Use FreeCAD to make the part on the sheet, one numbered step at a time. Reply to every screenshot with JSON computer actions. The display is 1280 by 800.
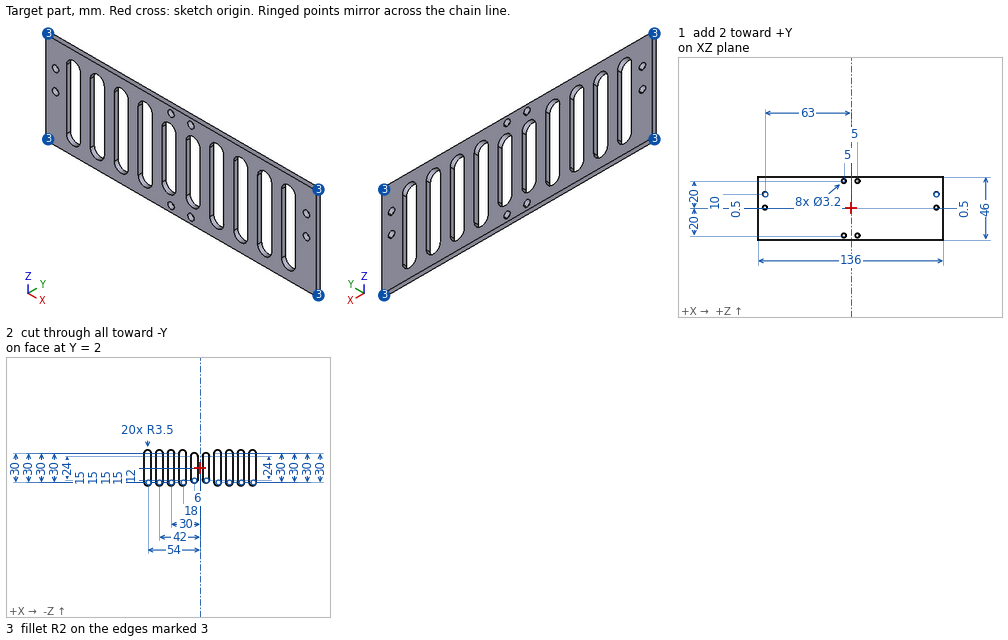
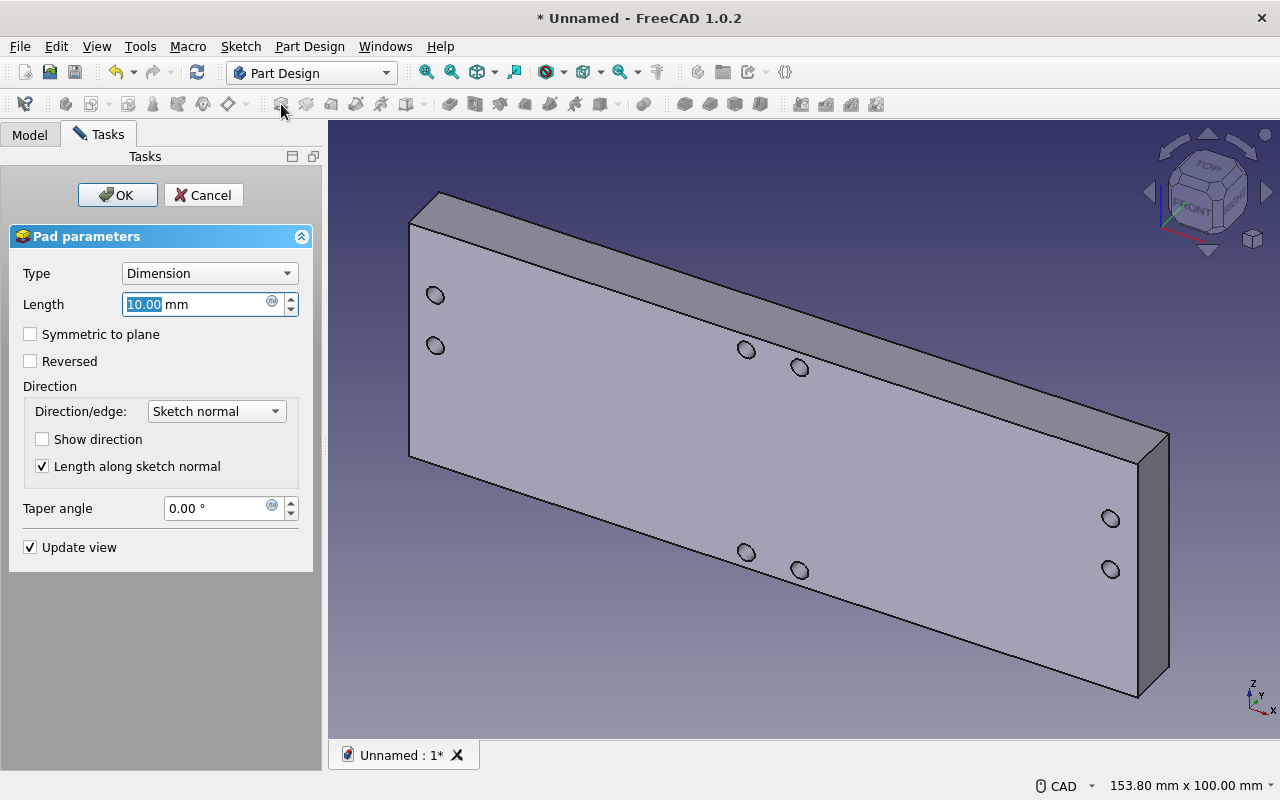
{"action": "type", "text": "2"}
{"action": "key", "text": "Tab"}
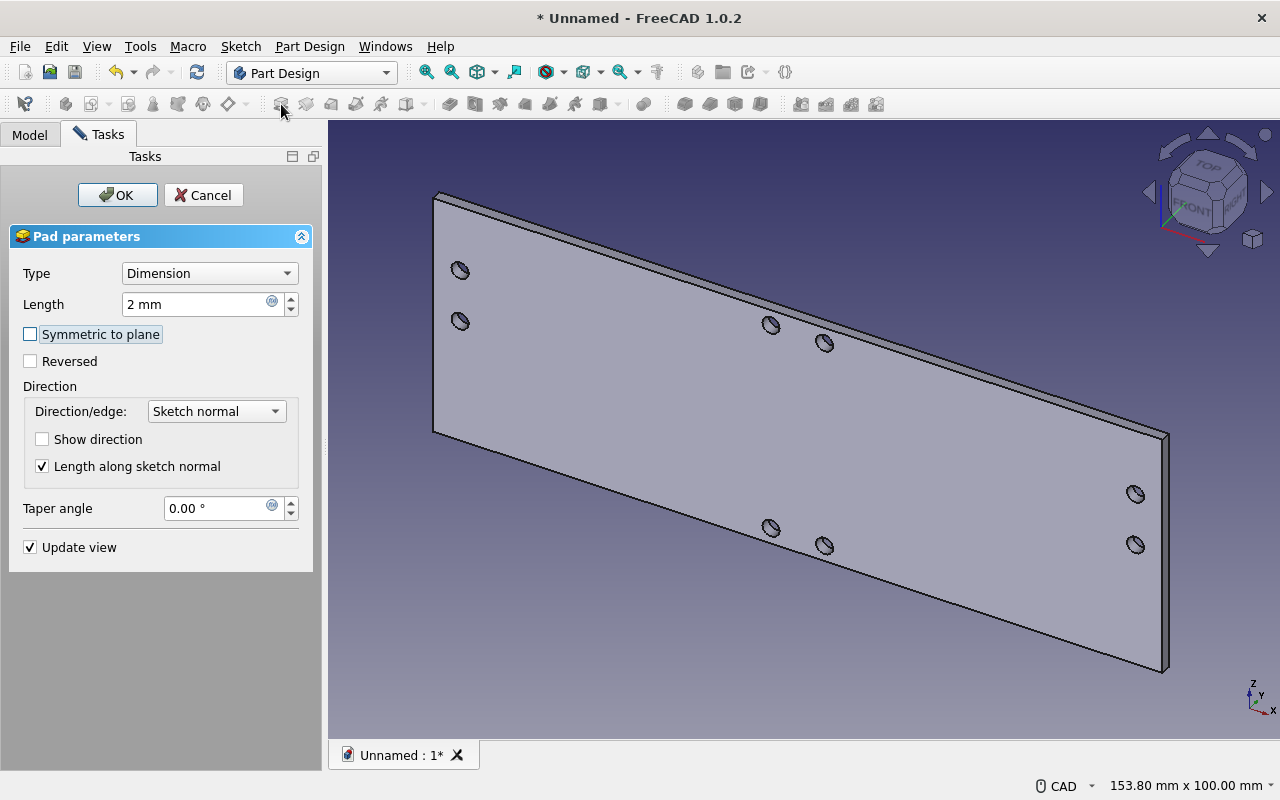
{"action": "left_click", "coordinate": [31, 361]}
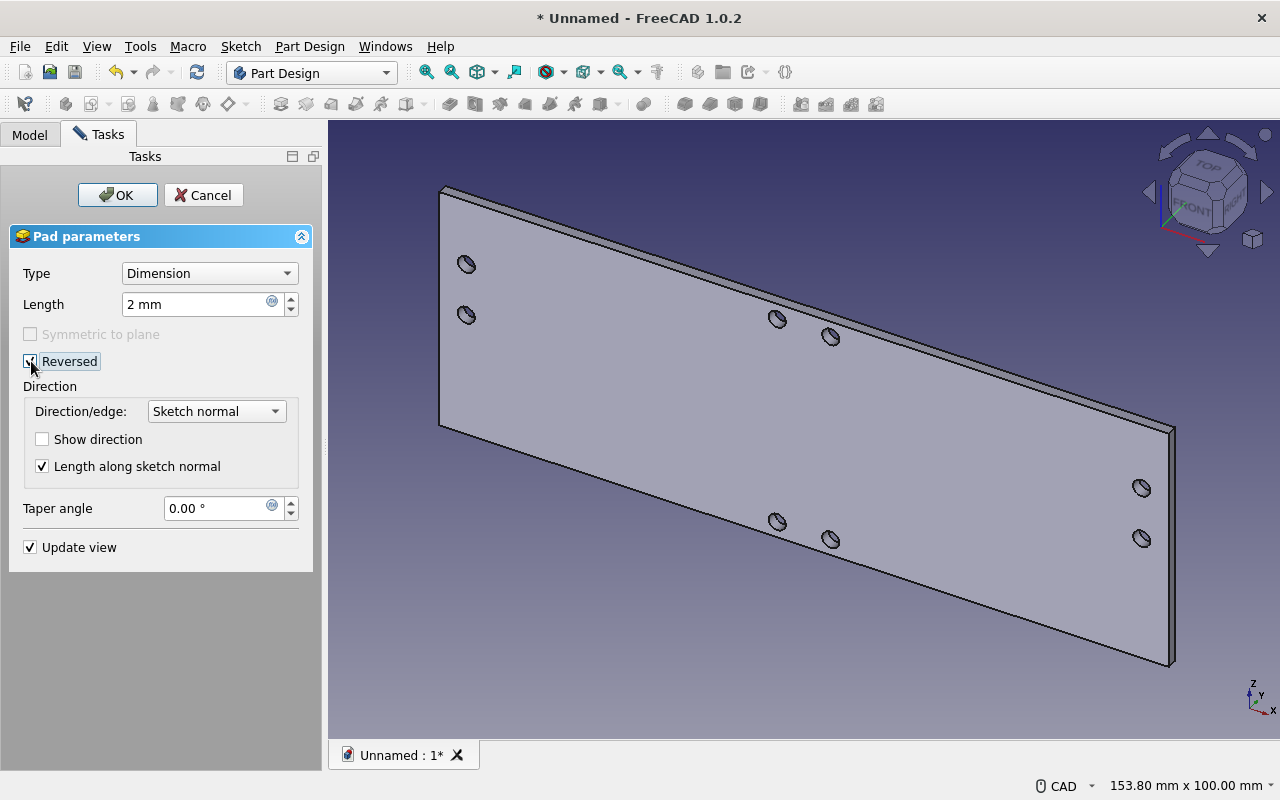
{"action": "left_click", "coordinate": [118, 195]}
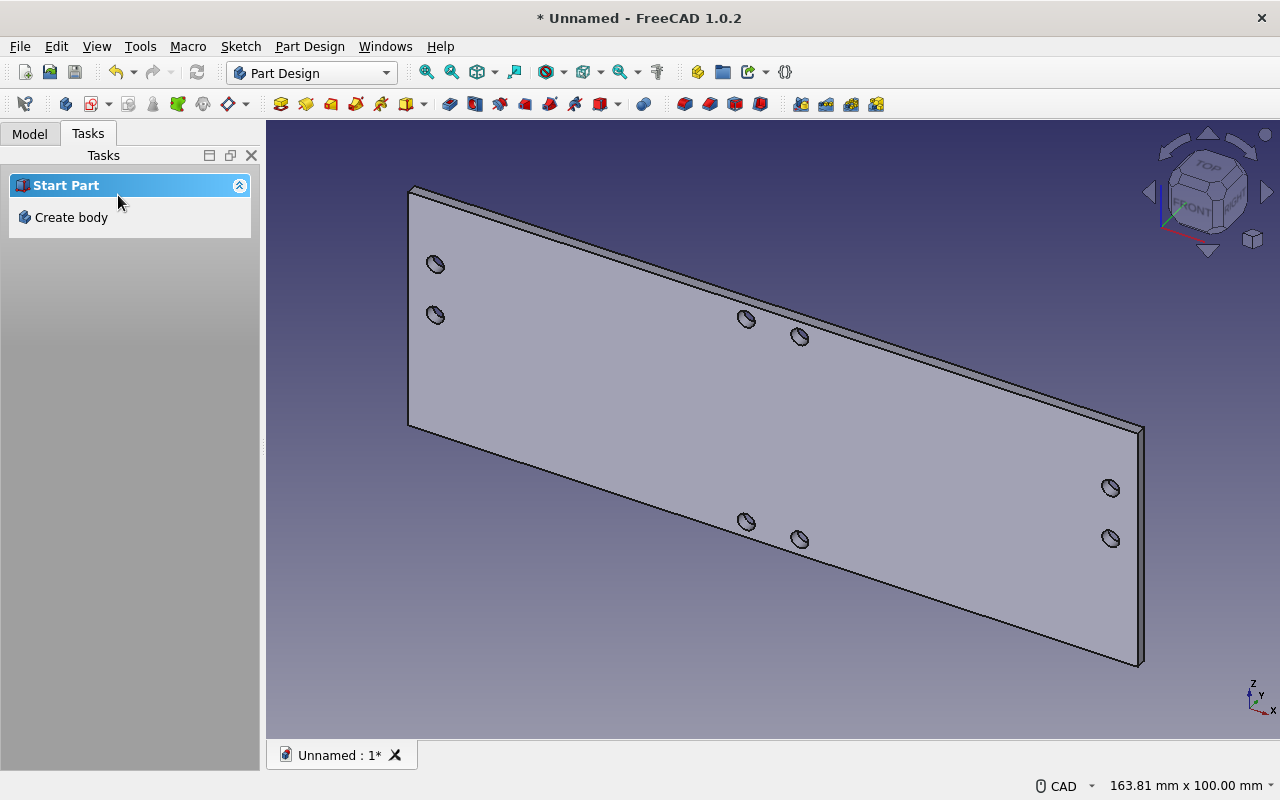
{"action": "key", "text": "4"}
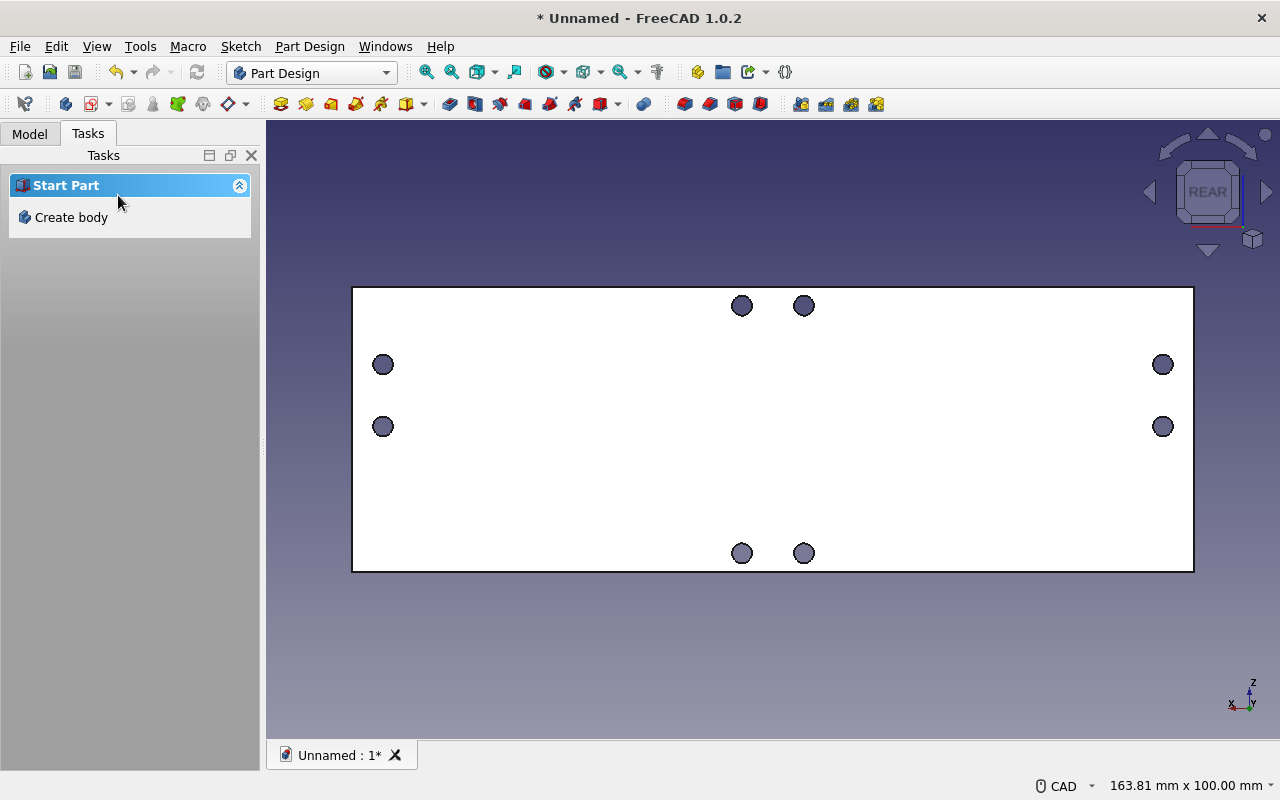
{"action": "left_click", "coordinate": [653, 428]}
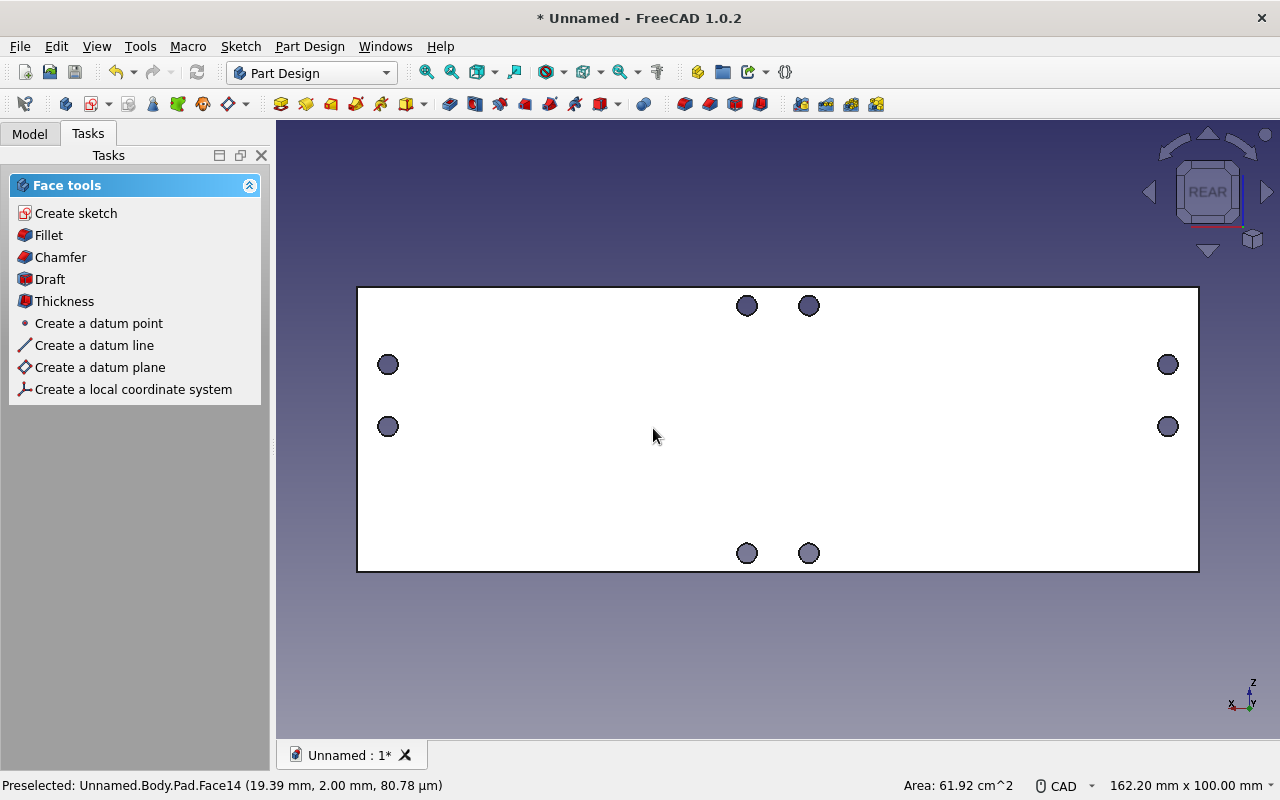
{"action": "left_click", "coordinate": [90, 104]}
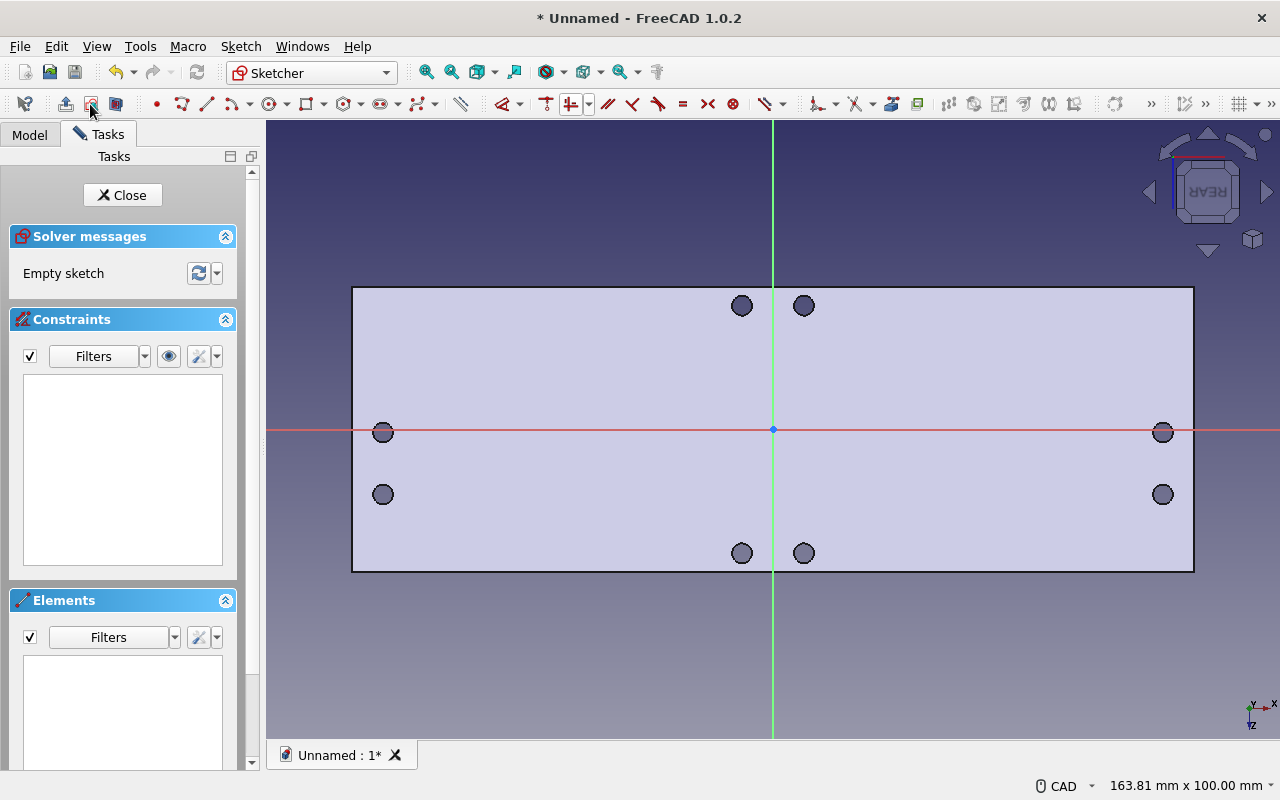
{"action": "scroll", "coordinate": [395, 429], "scroll_direction": "down", "scroll_amount": 1}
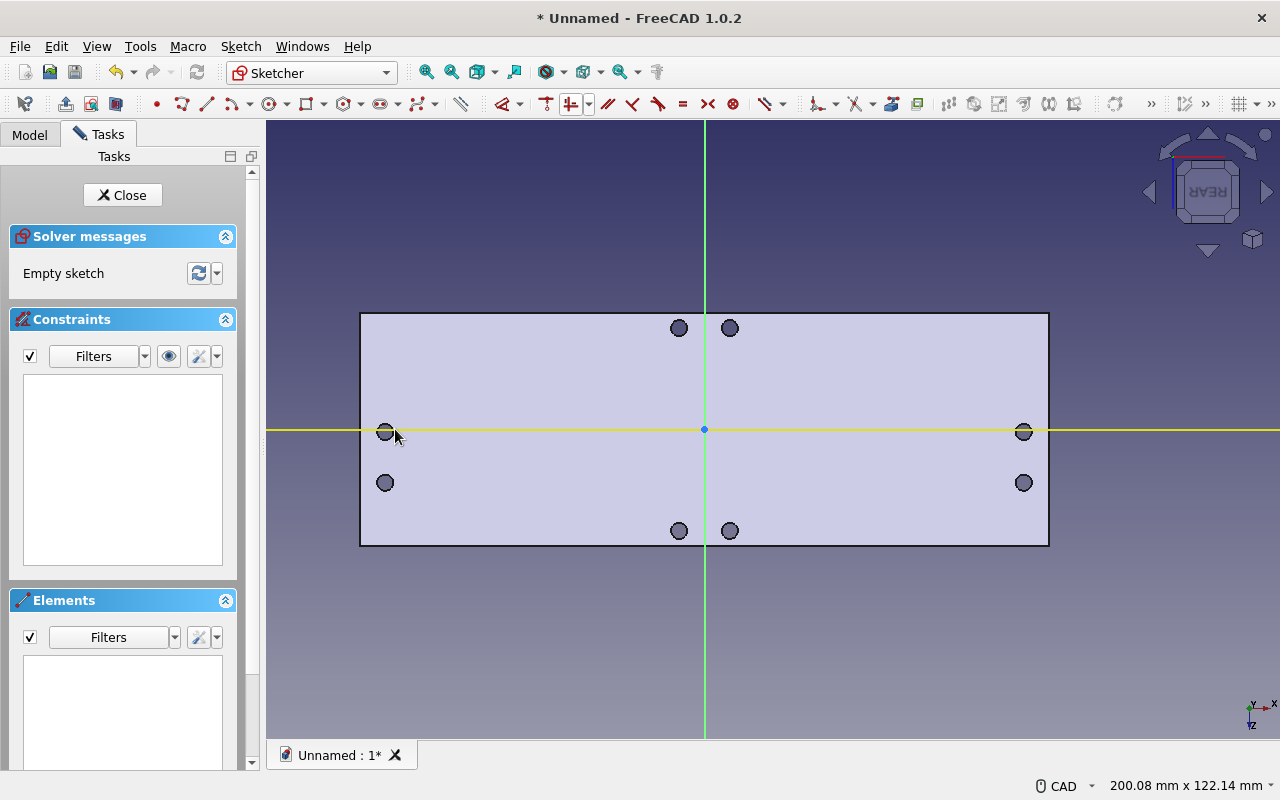
{"action": "left_click", "coordinate": [380, 104]}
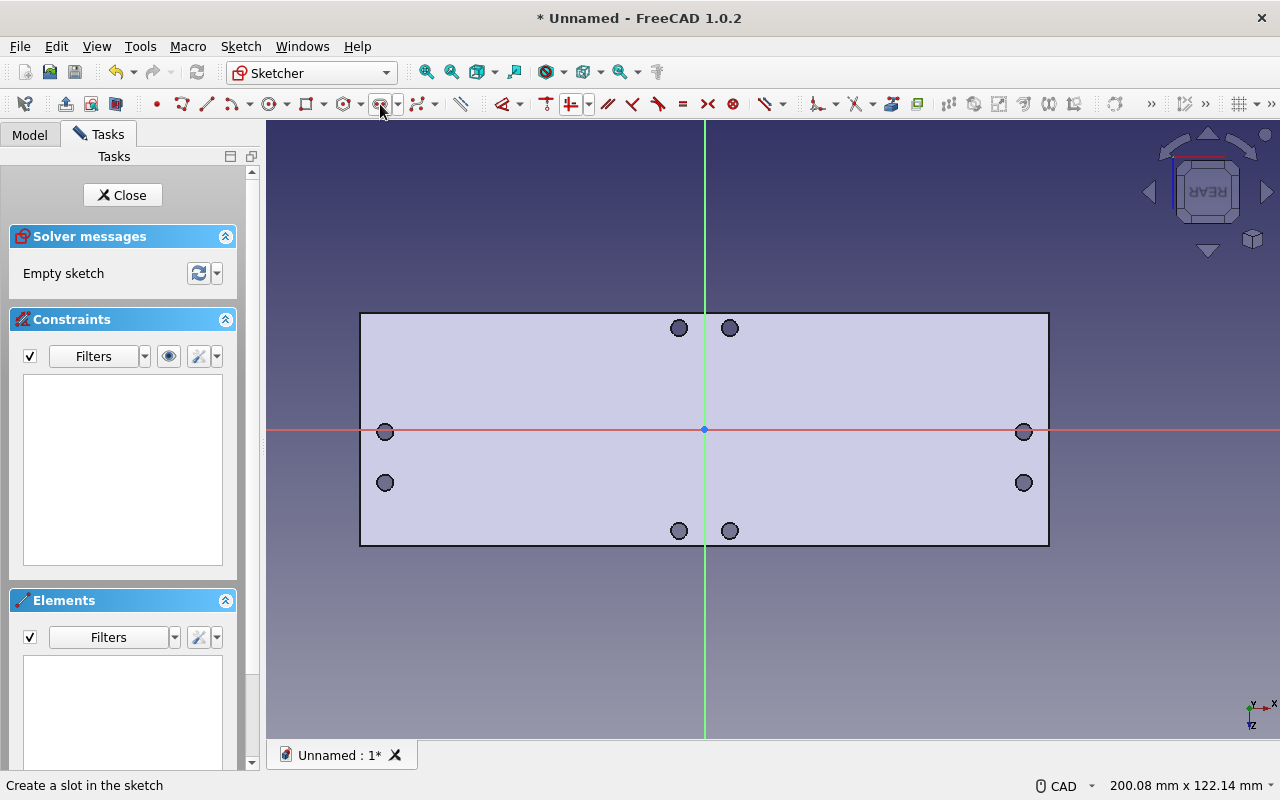
{"action": "scroll", "coordinate": [431, 506], "scroll_direction": "up", "scroll_amount": 2}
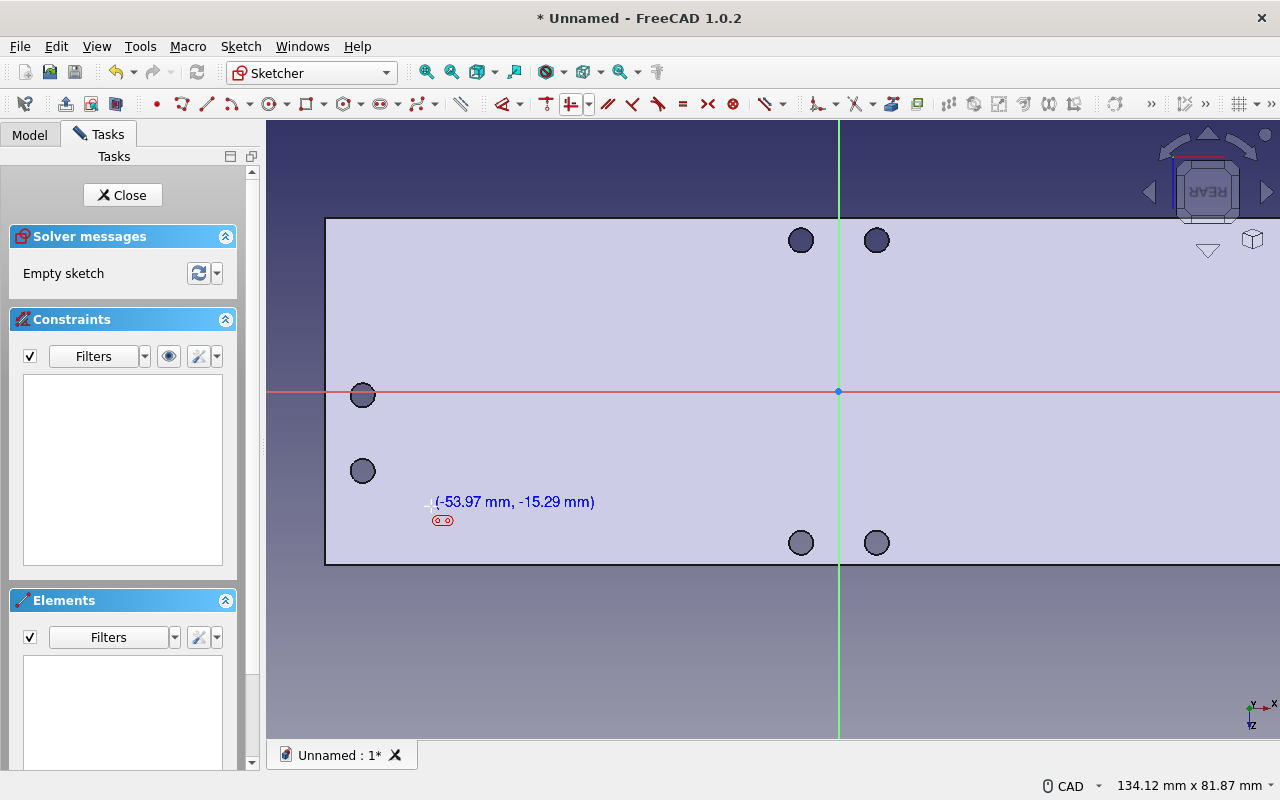
{"action": "left_click", "coordinate": [431, 505]}